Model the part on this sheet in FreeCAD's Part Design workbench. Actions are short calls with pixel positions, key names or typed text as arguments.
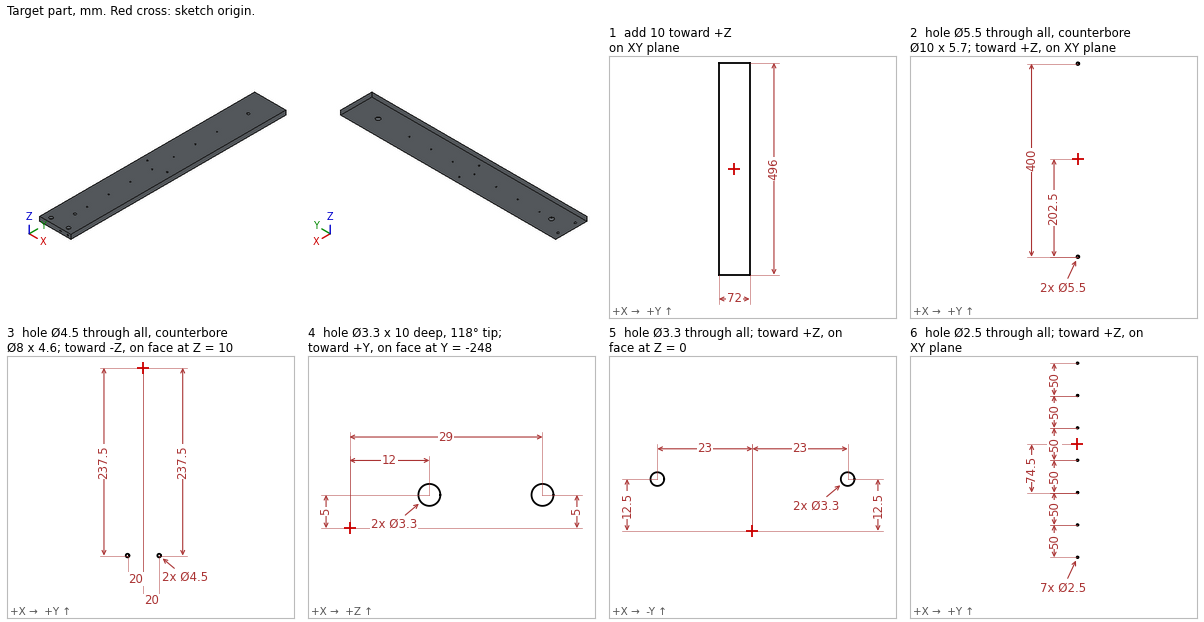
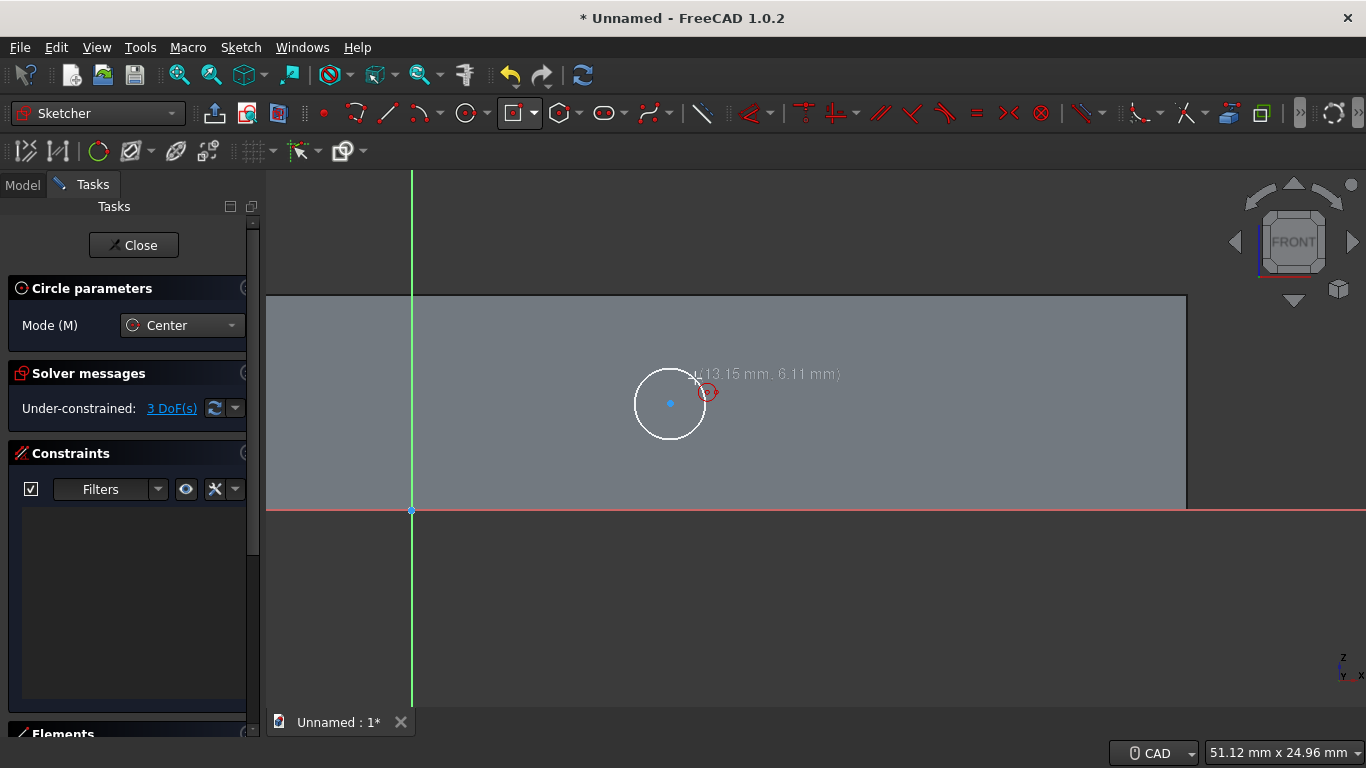
click(1036, 403)
click(1061, 378)
key(Escape)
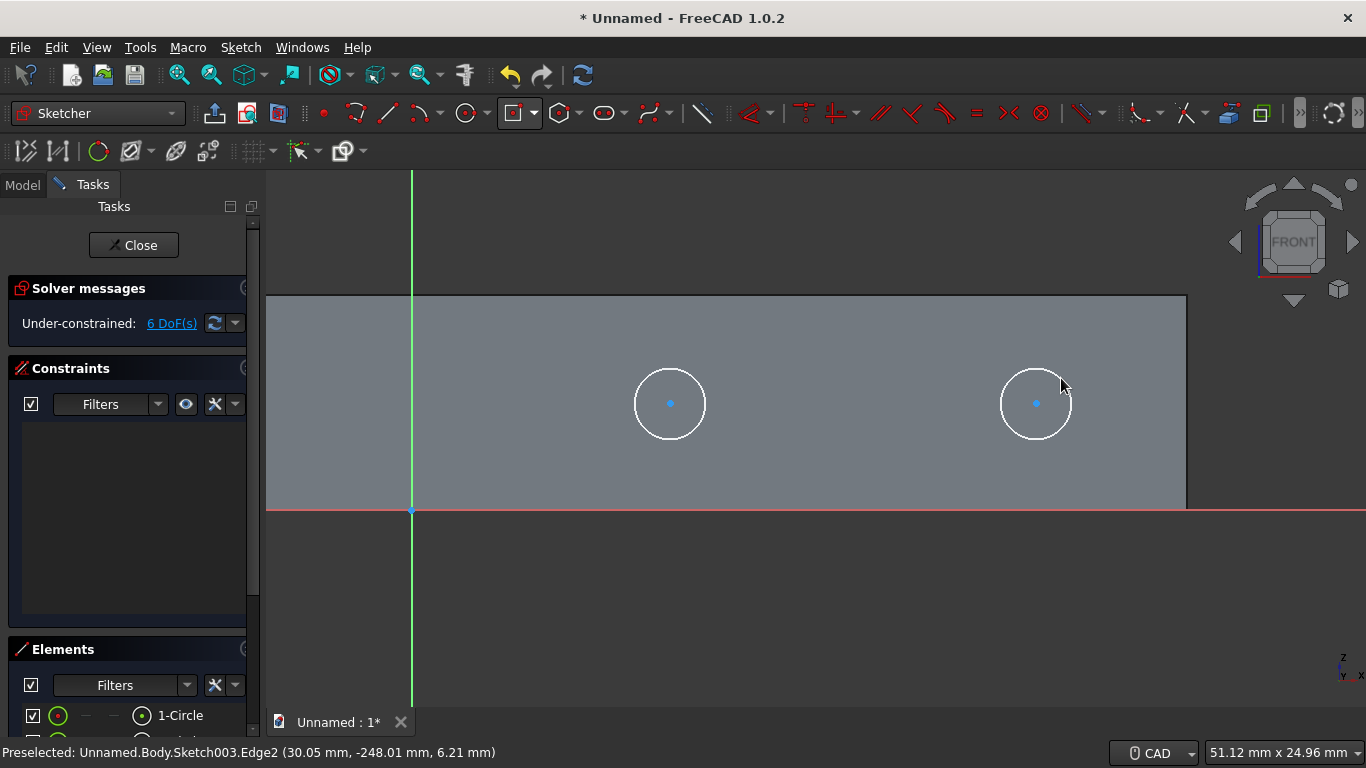
click(695, 379)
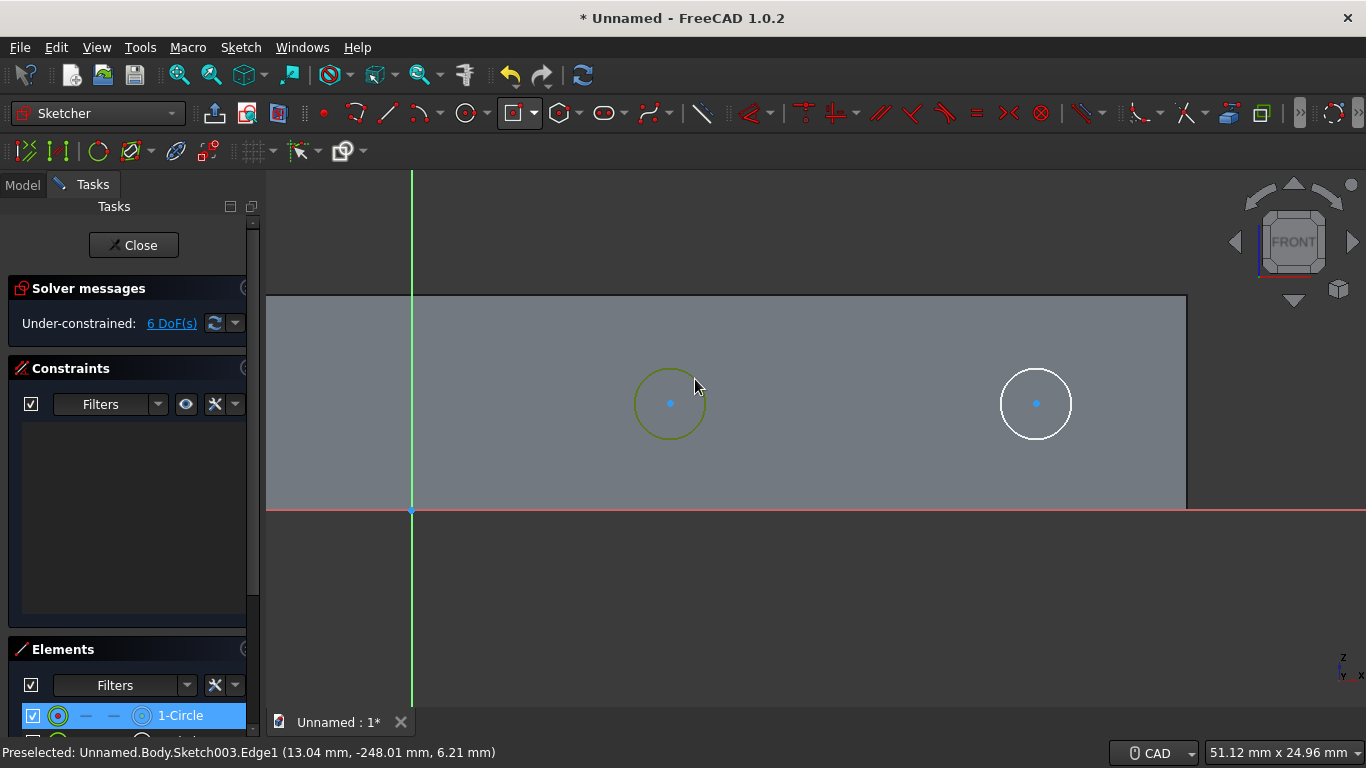
click(1061, 379)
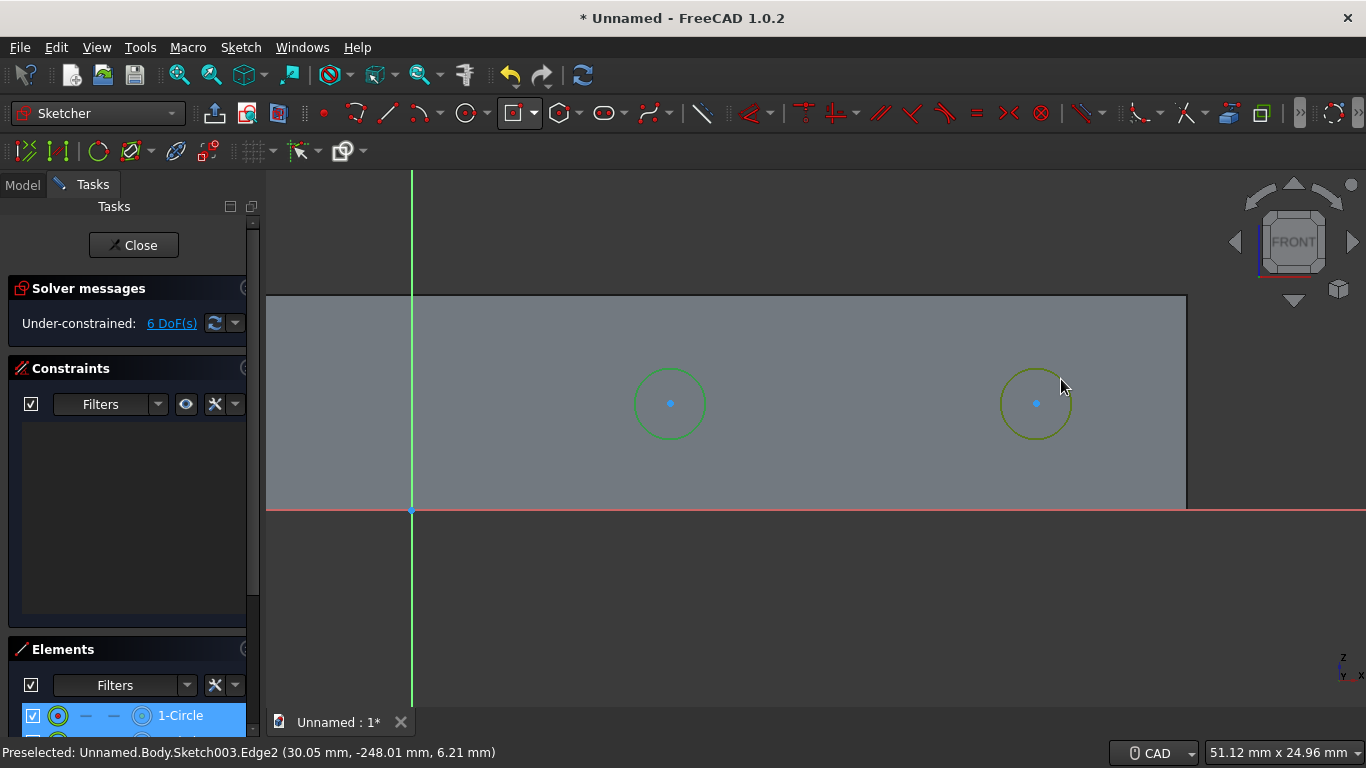
click(978, 114)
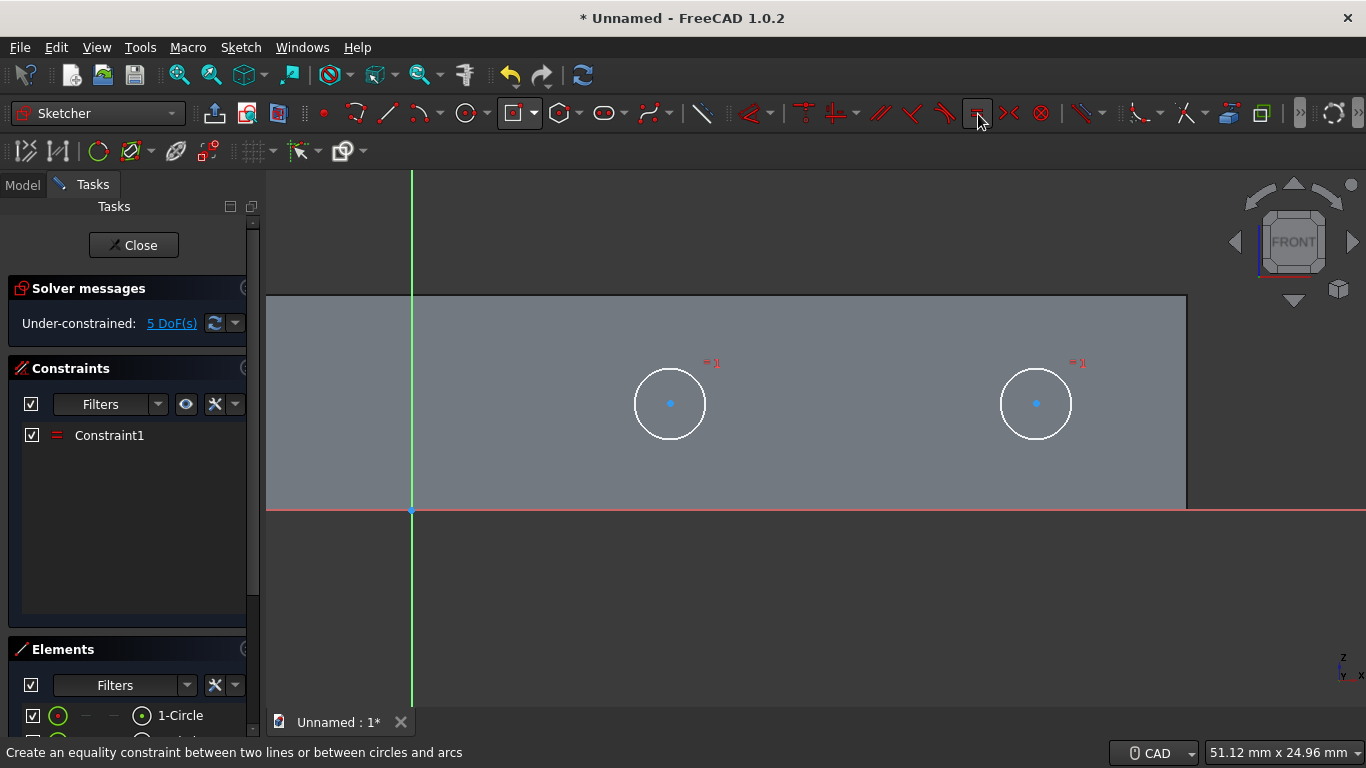
click(750, 114)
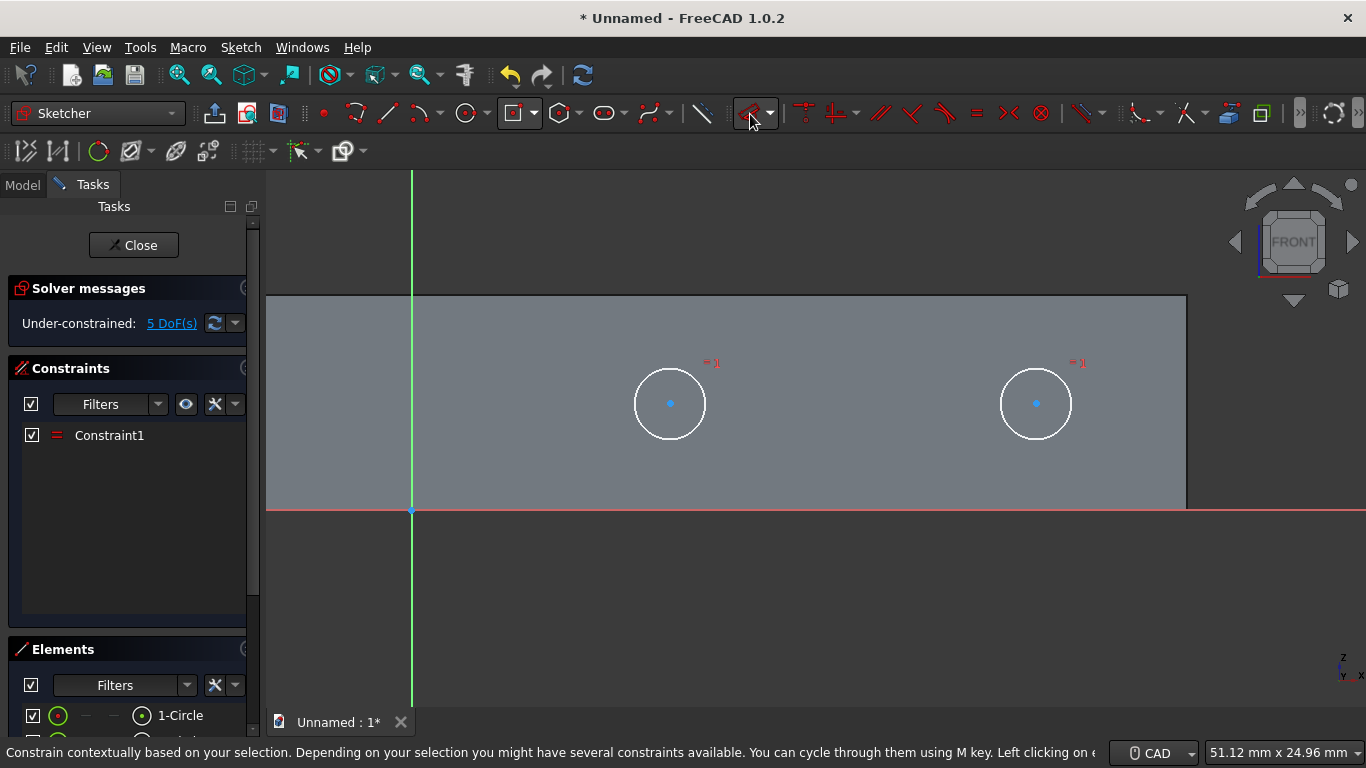
click(695, 379)
click(718, 356)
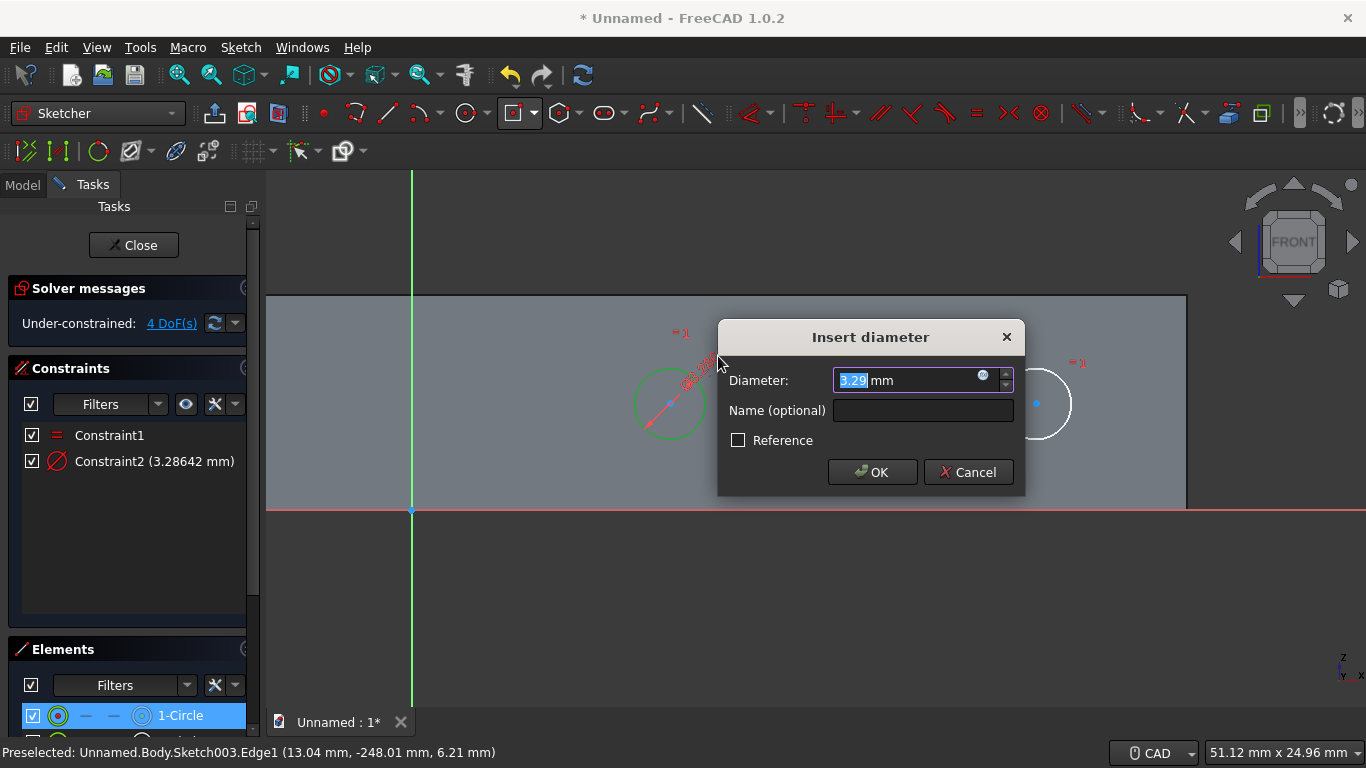
text(3.3)
key(Return)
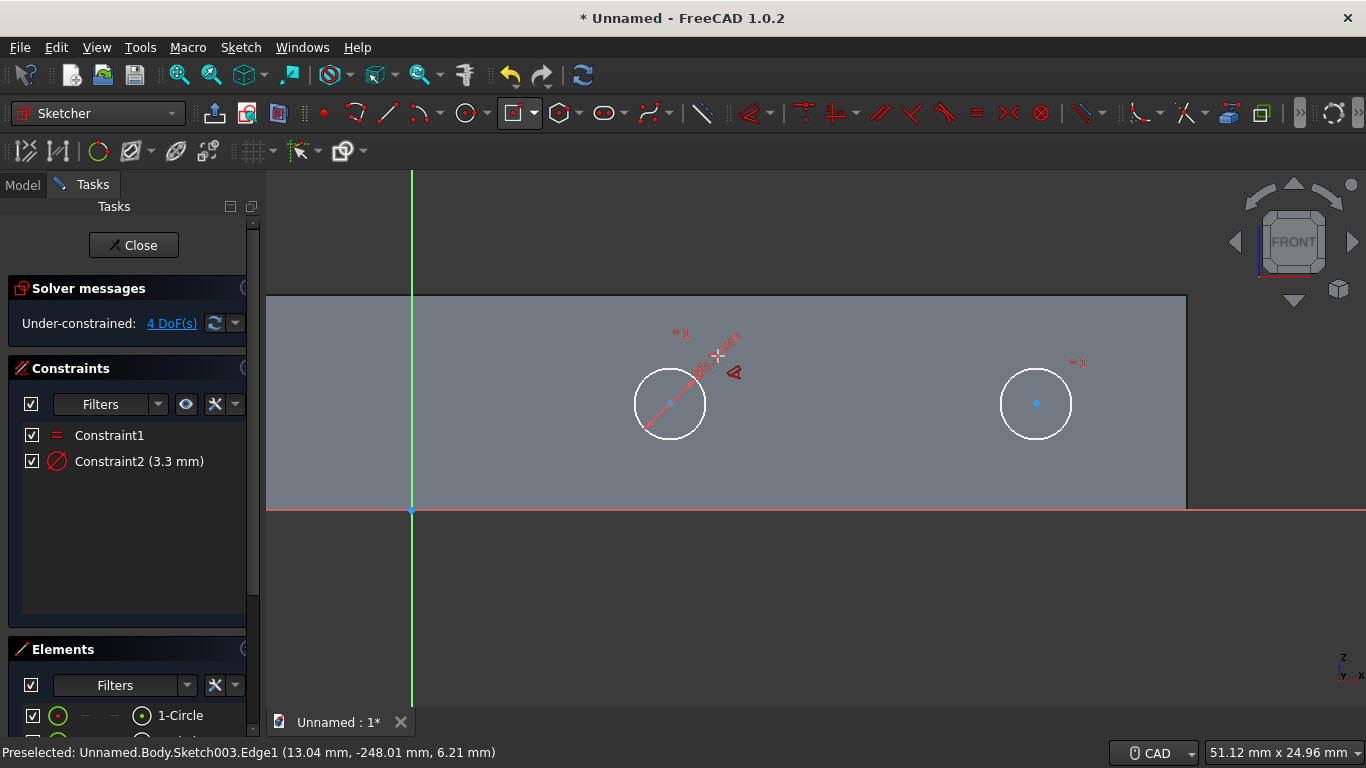
click(670, 404)
click(378, 457)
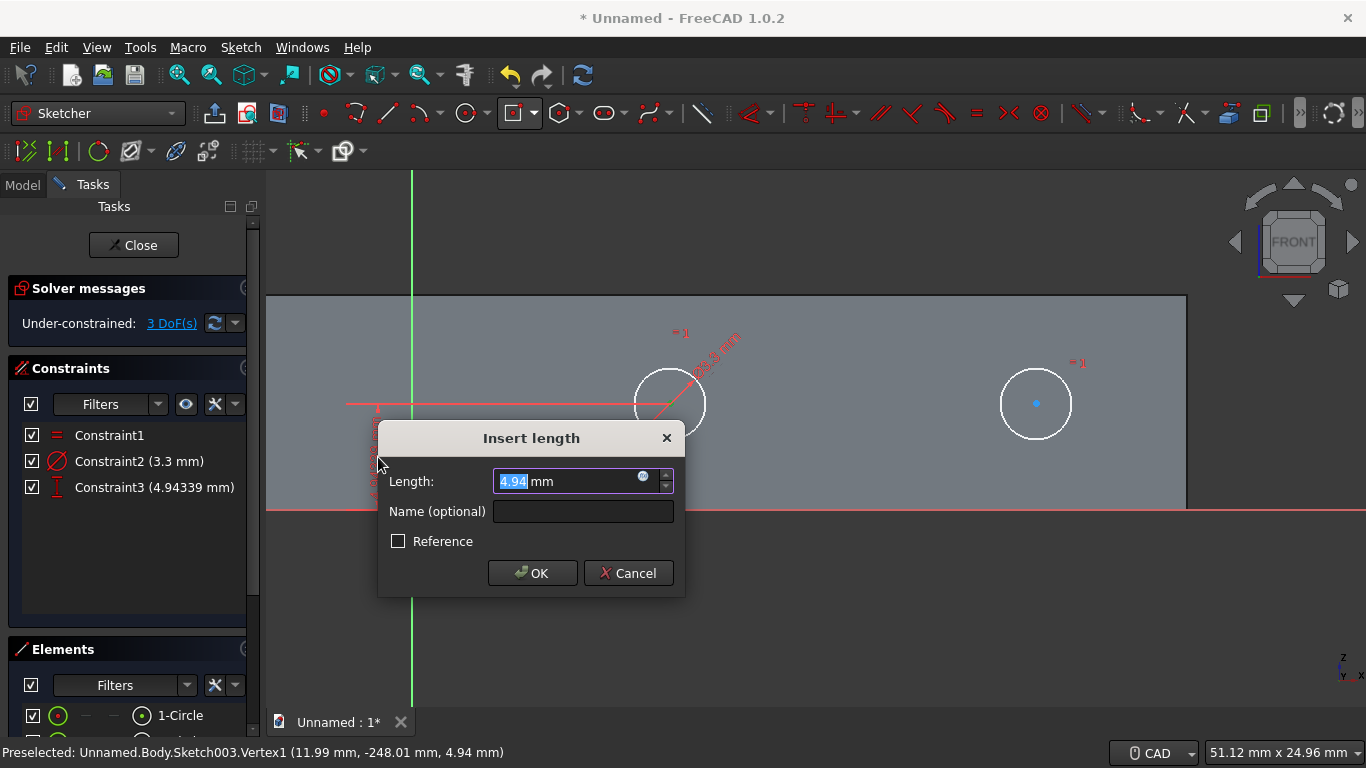
text(5)
key(Return)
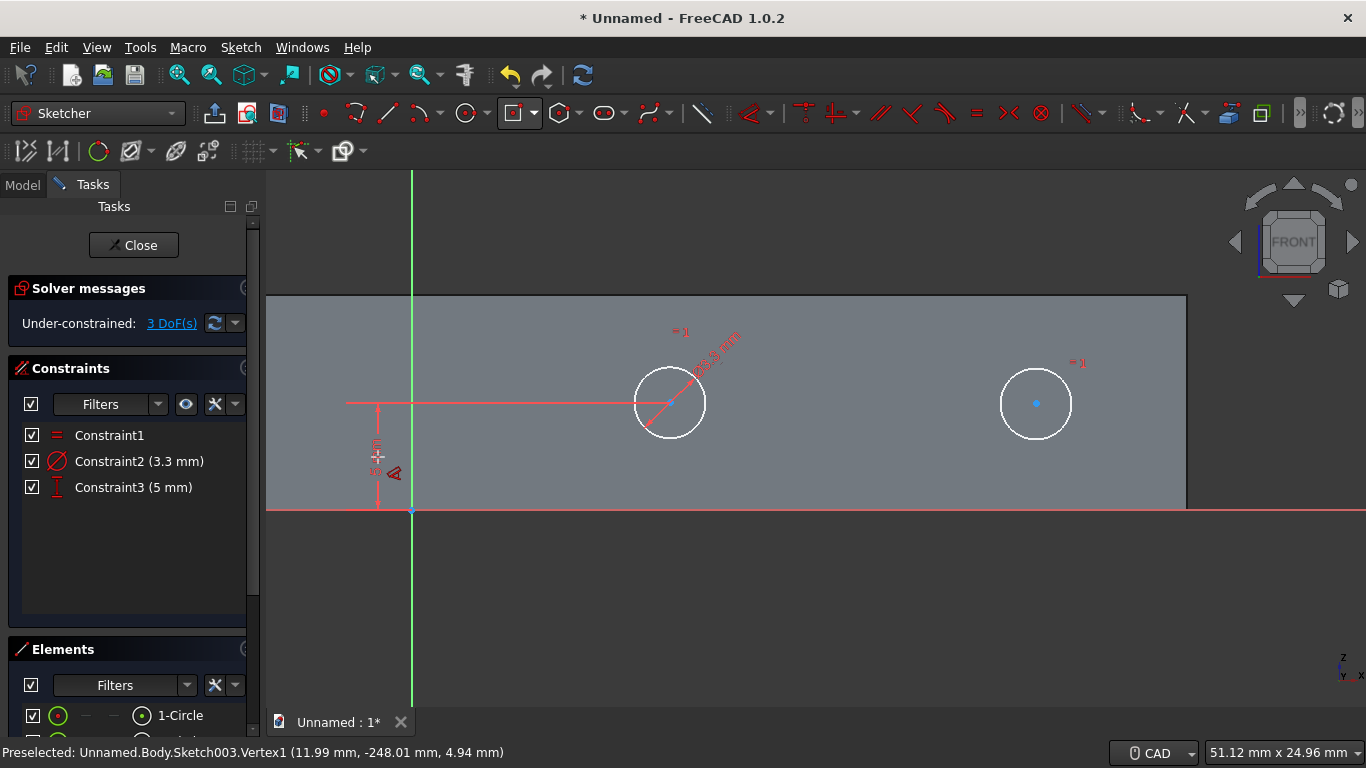
click(1036, 404)
click(378, 433)